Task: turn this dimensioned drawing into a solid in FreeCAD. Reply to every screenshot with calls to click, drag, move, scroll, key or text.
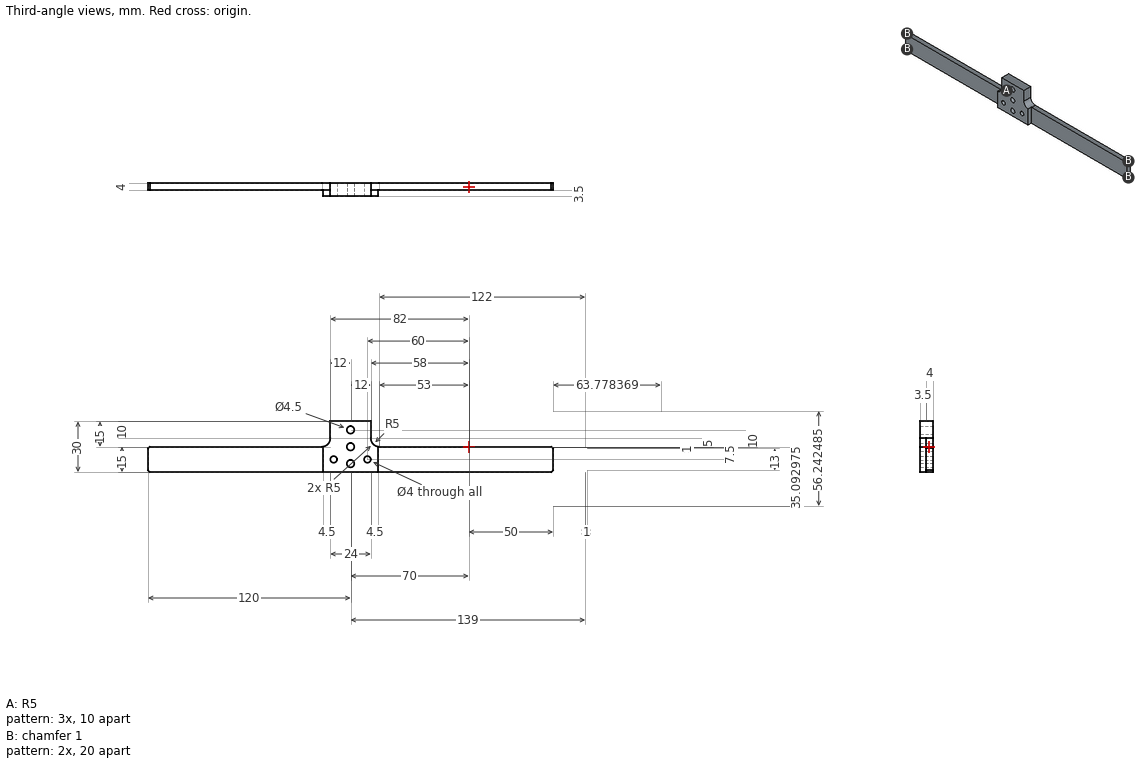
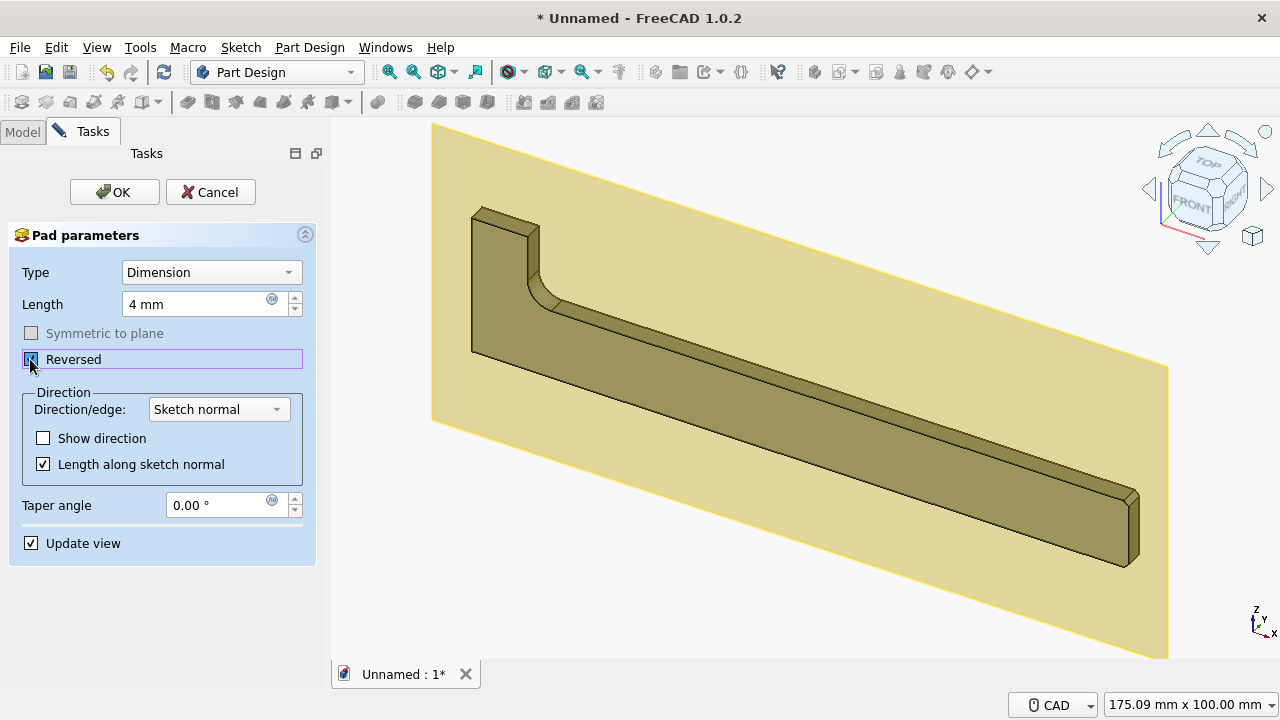
click(115, 192)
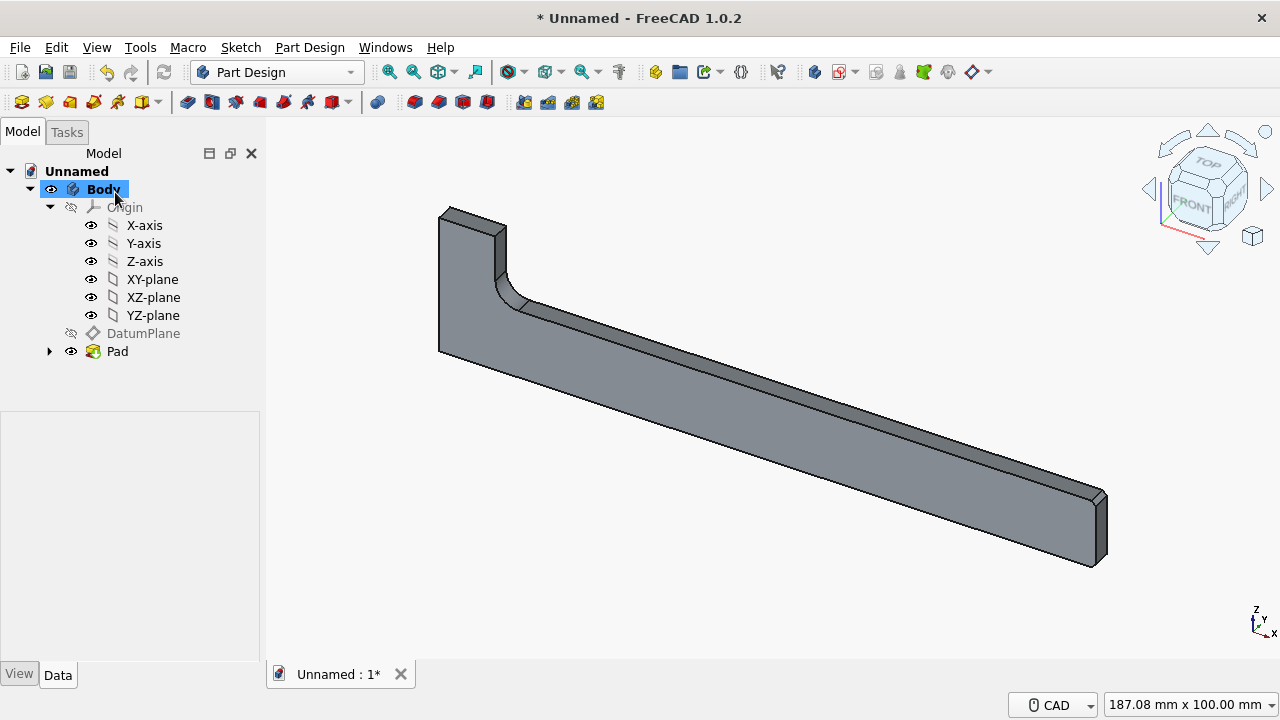
key(4)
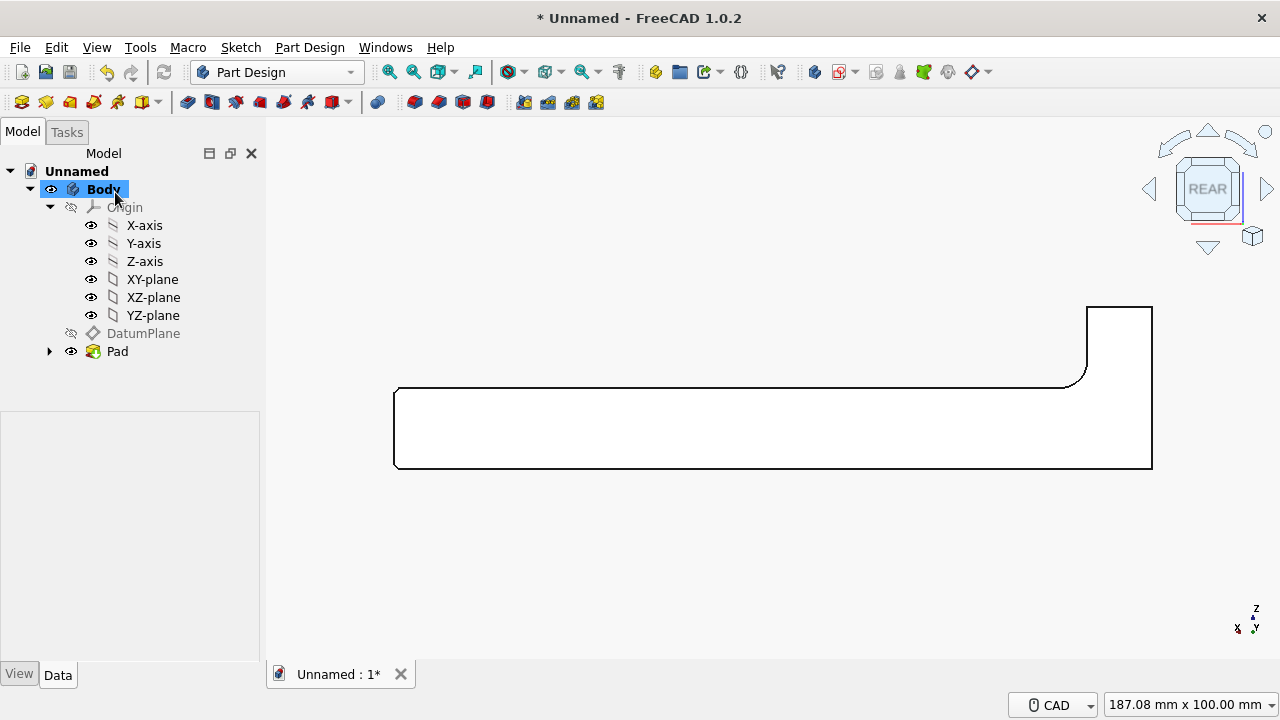
click(1098, 410)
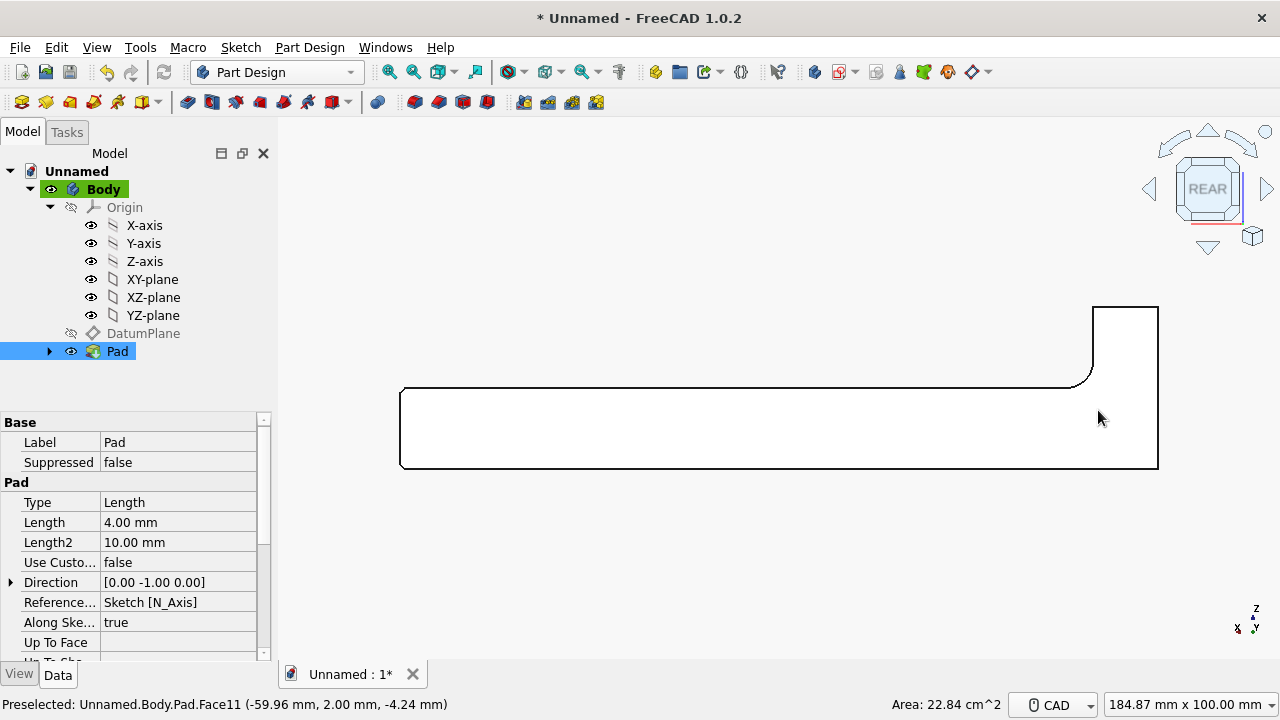
click(840, 72)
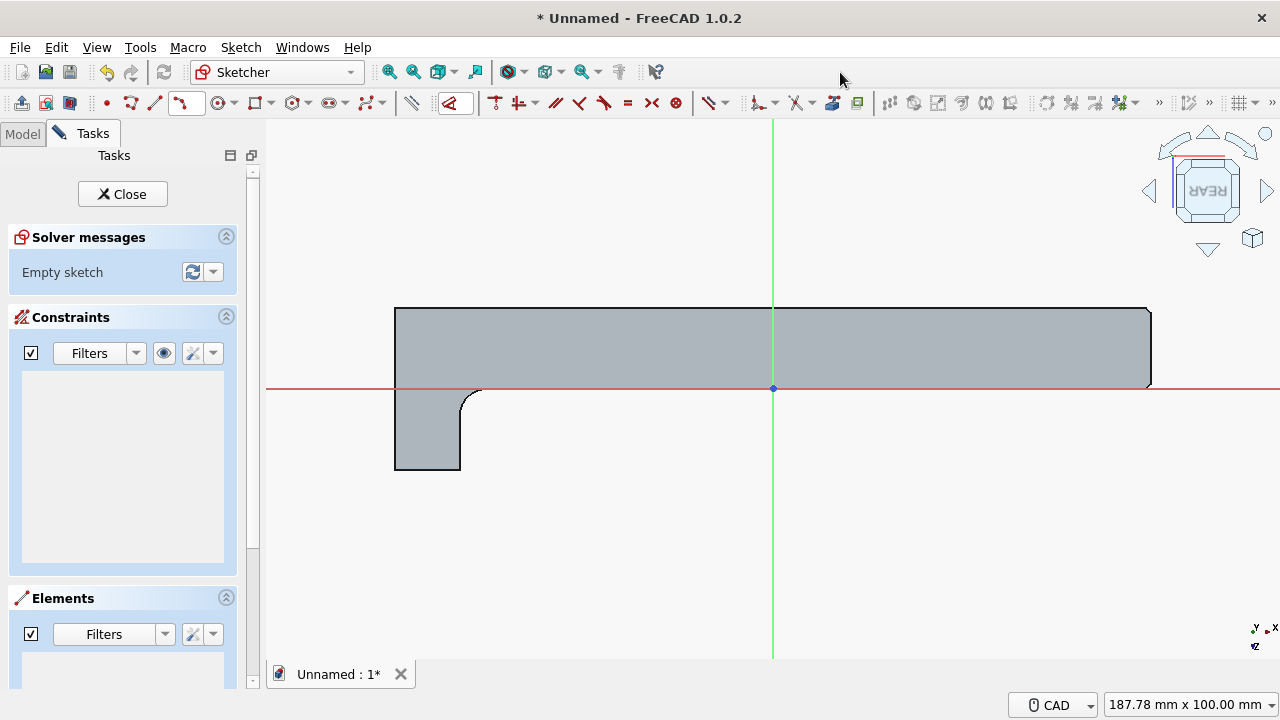
scroll(1115, 389, down, 3)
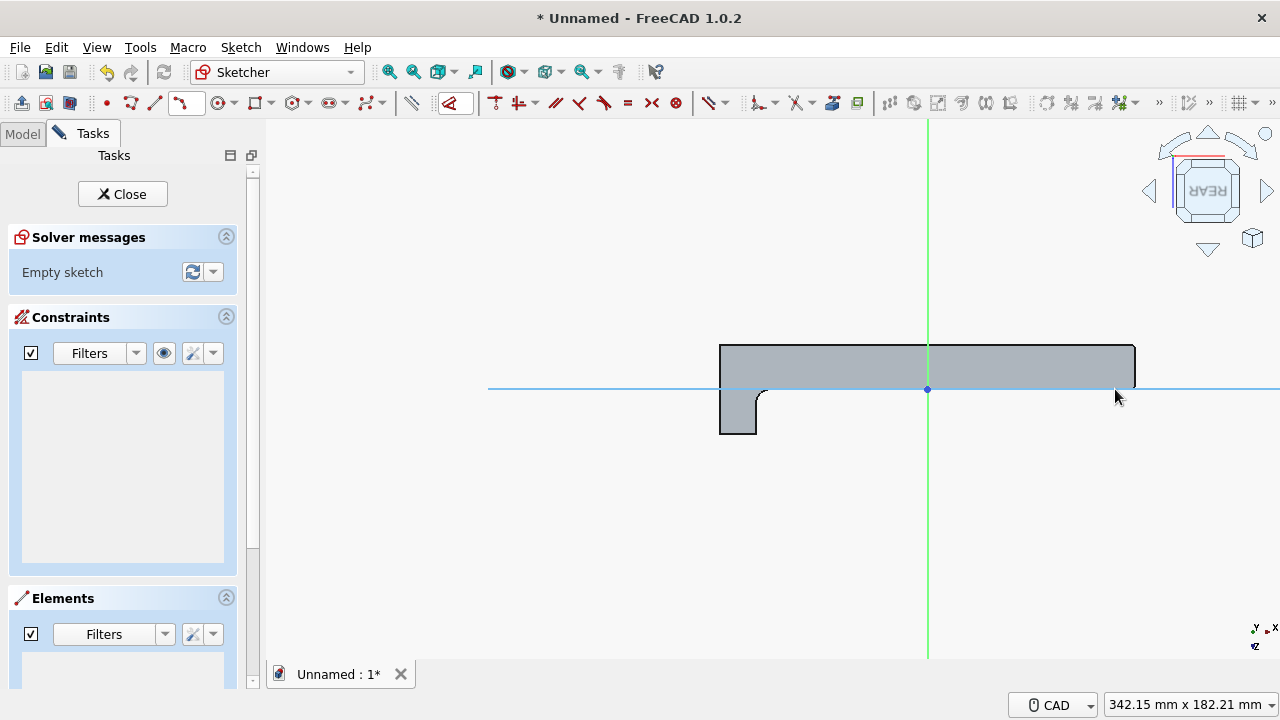
click(132, 104)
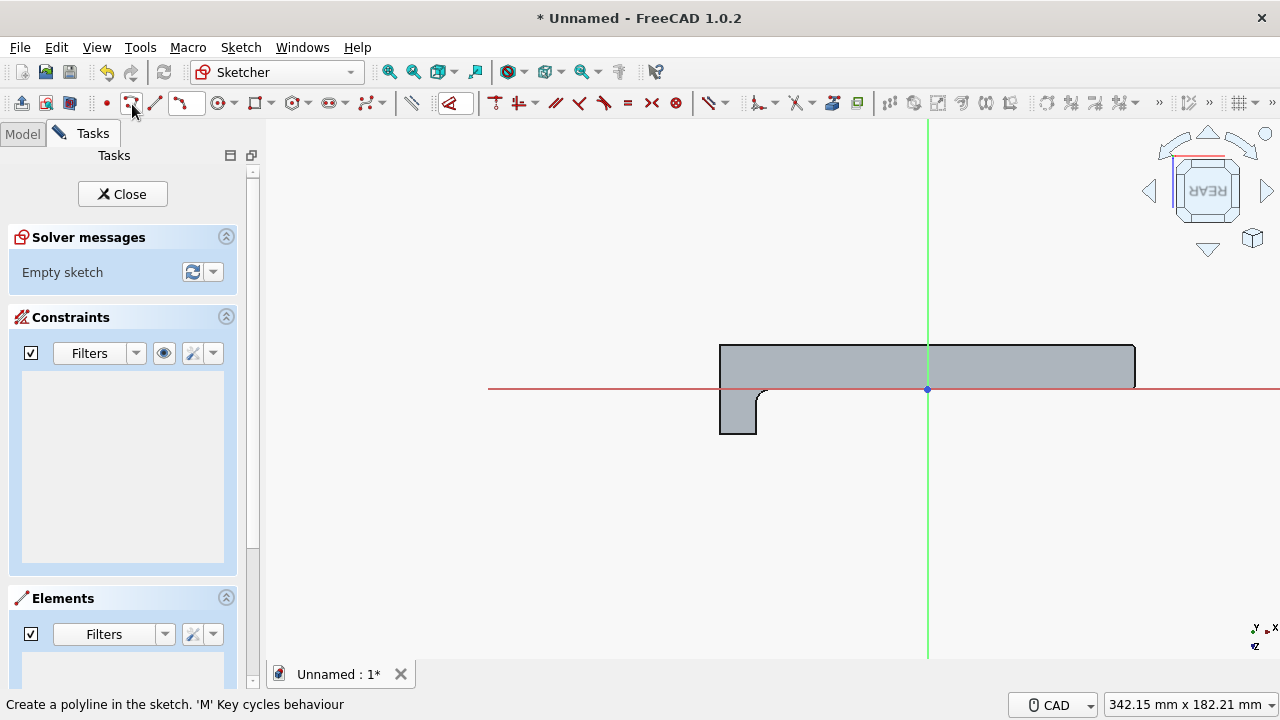
click(720, 345)
click(365, 345)
click(365, 389)
click(685, 380)
click(685, 434)
click(720, 434)
click(720, 346)
key(Escape)
key(Escape)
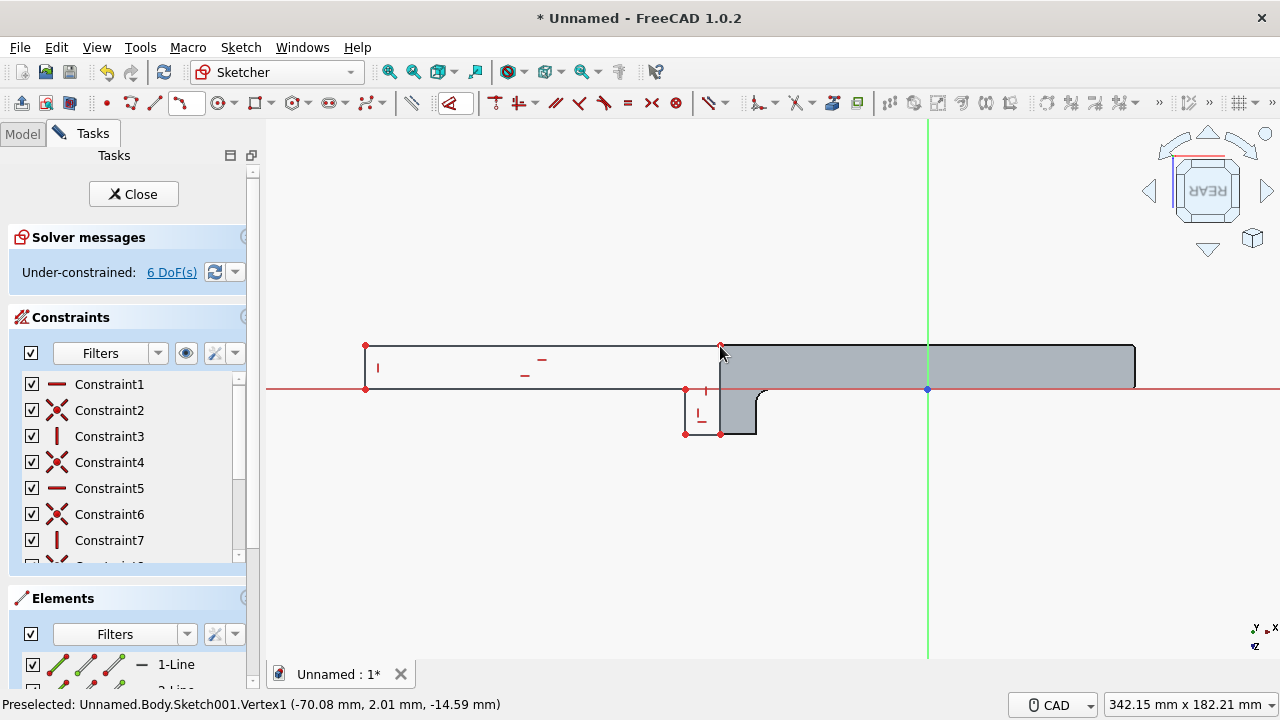
click(365, 389)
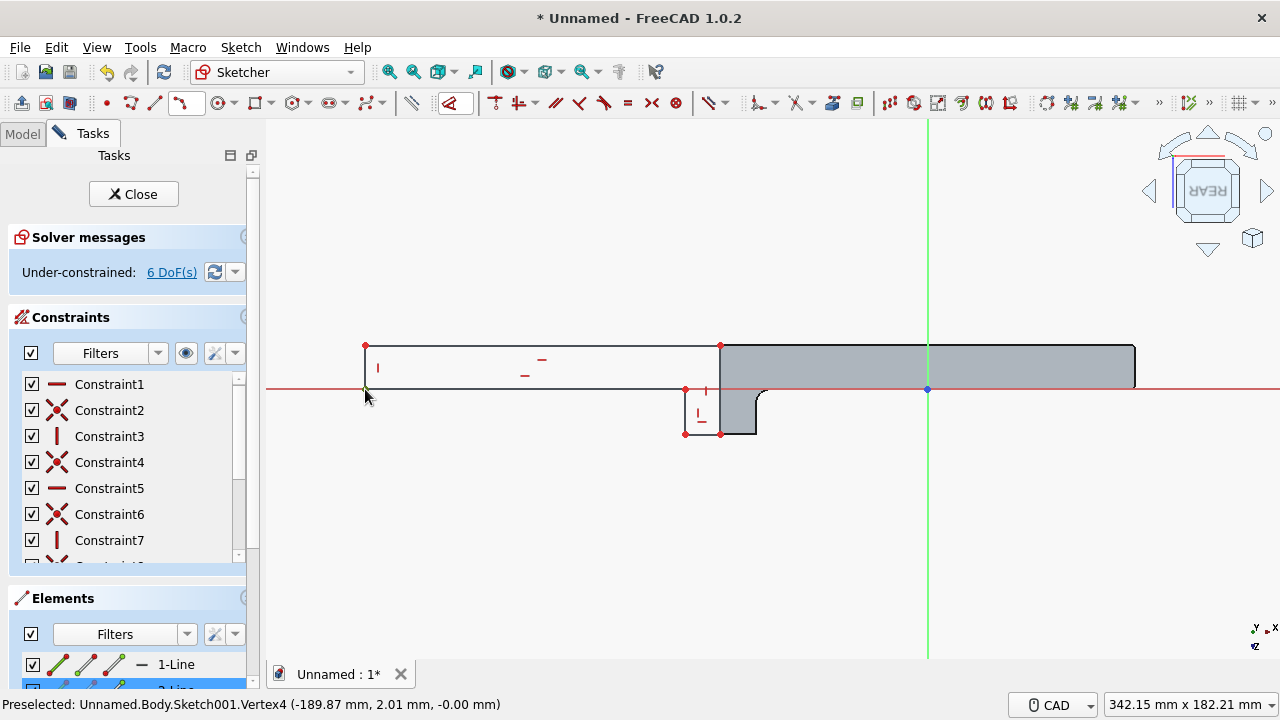
click(763, 389)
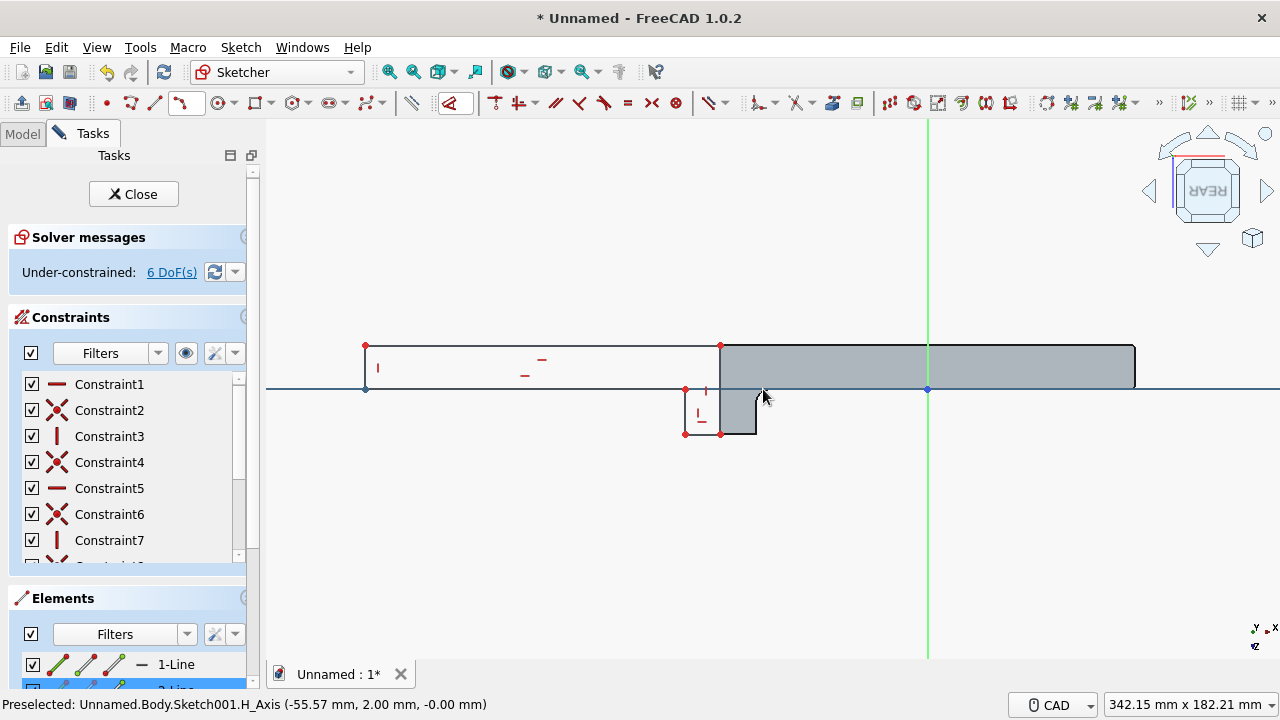
click(496, 104)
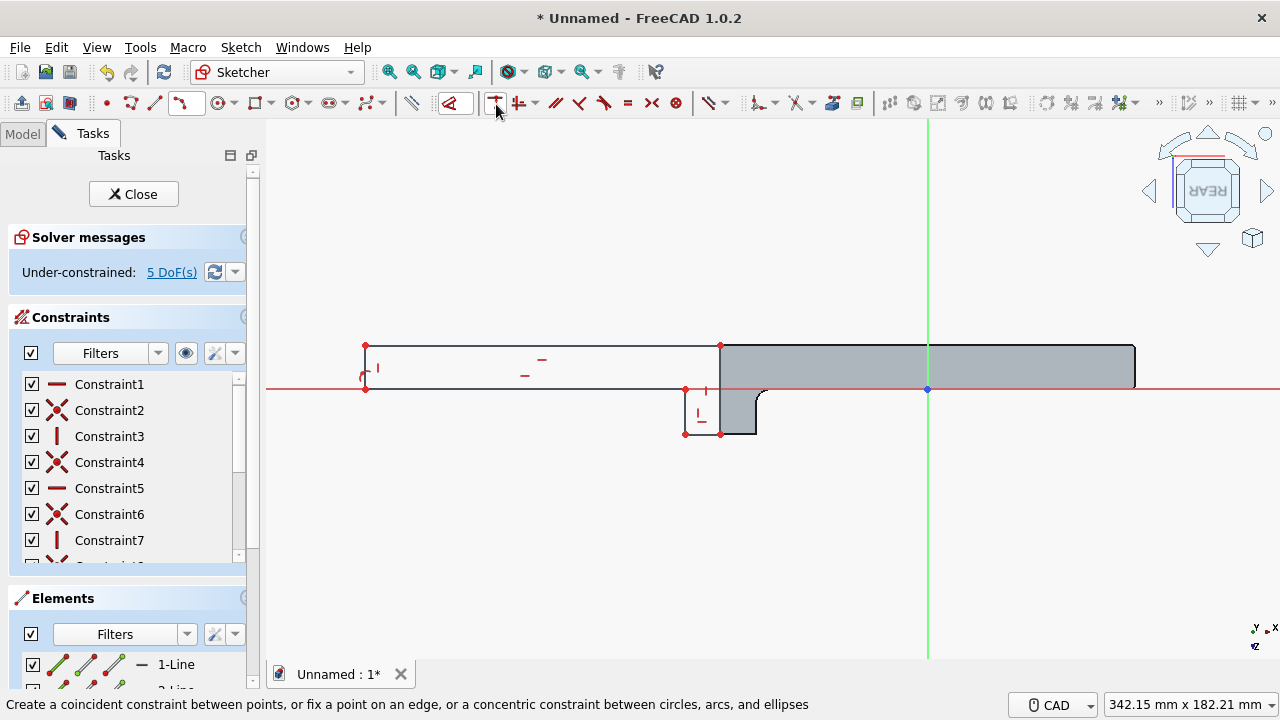
click(365, 359)